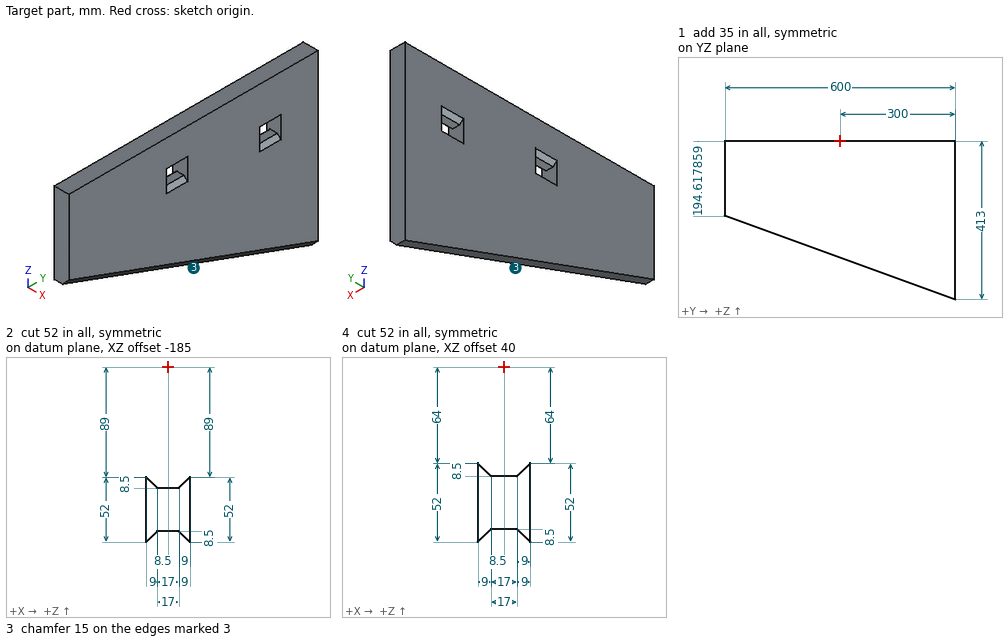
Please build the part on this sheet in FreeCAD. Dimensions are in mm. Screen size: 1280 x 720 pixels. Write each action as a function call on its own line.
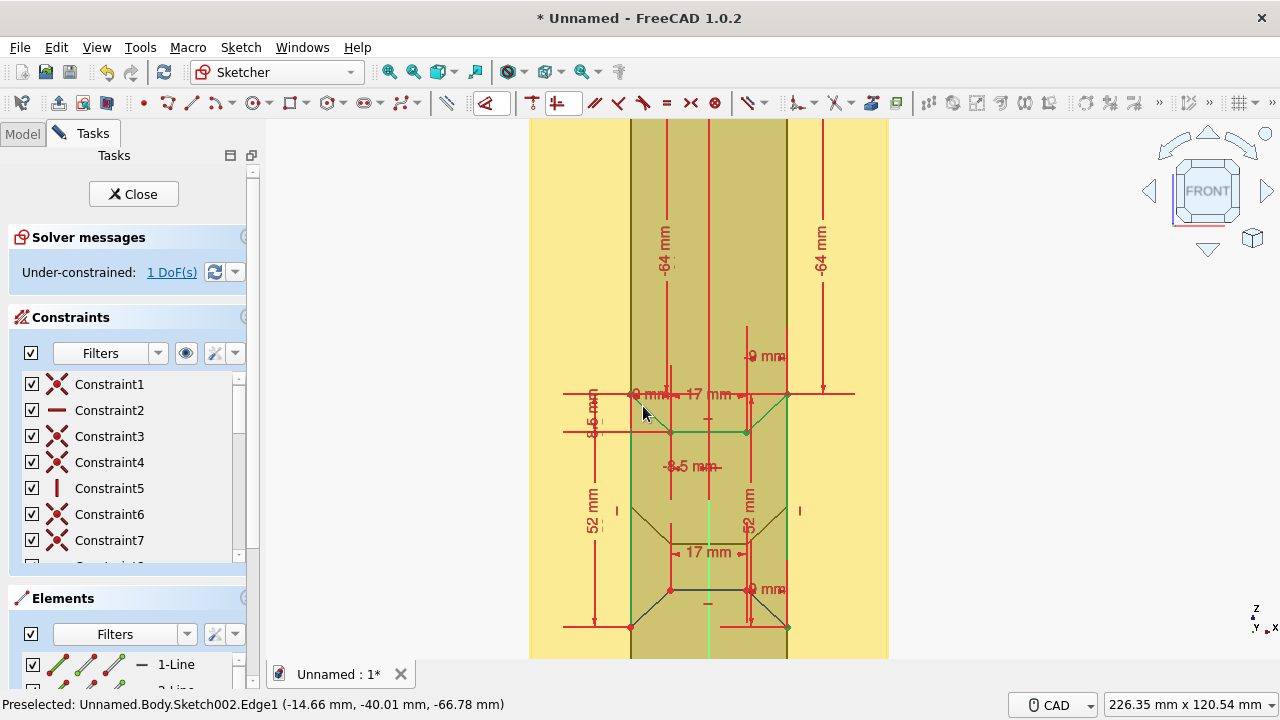
click(775, 616)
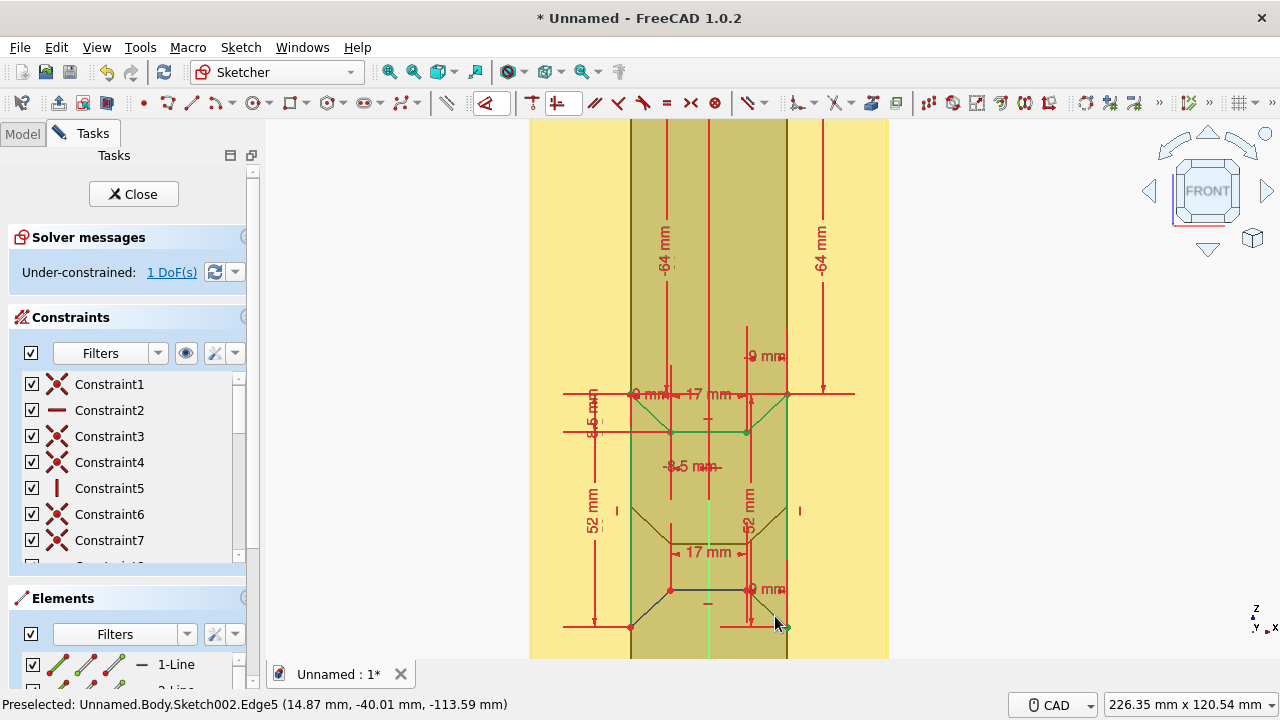
key(i)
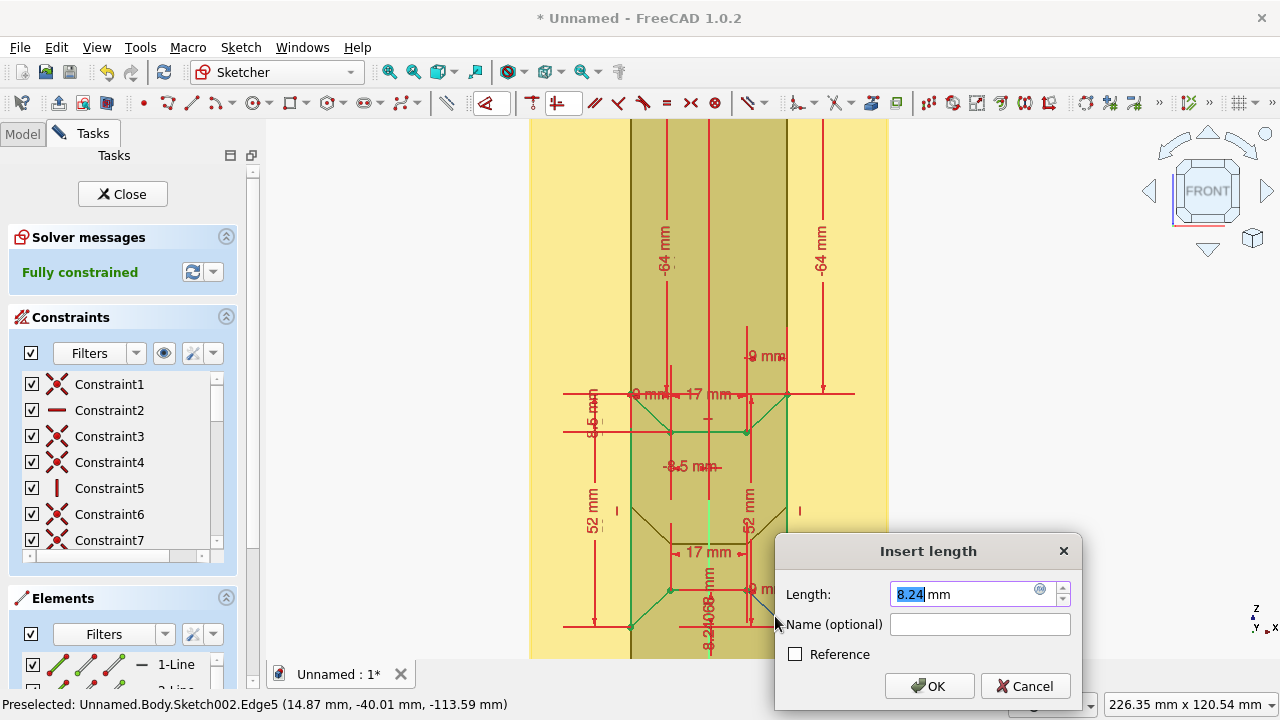
text(8.5)
key(Return)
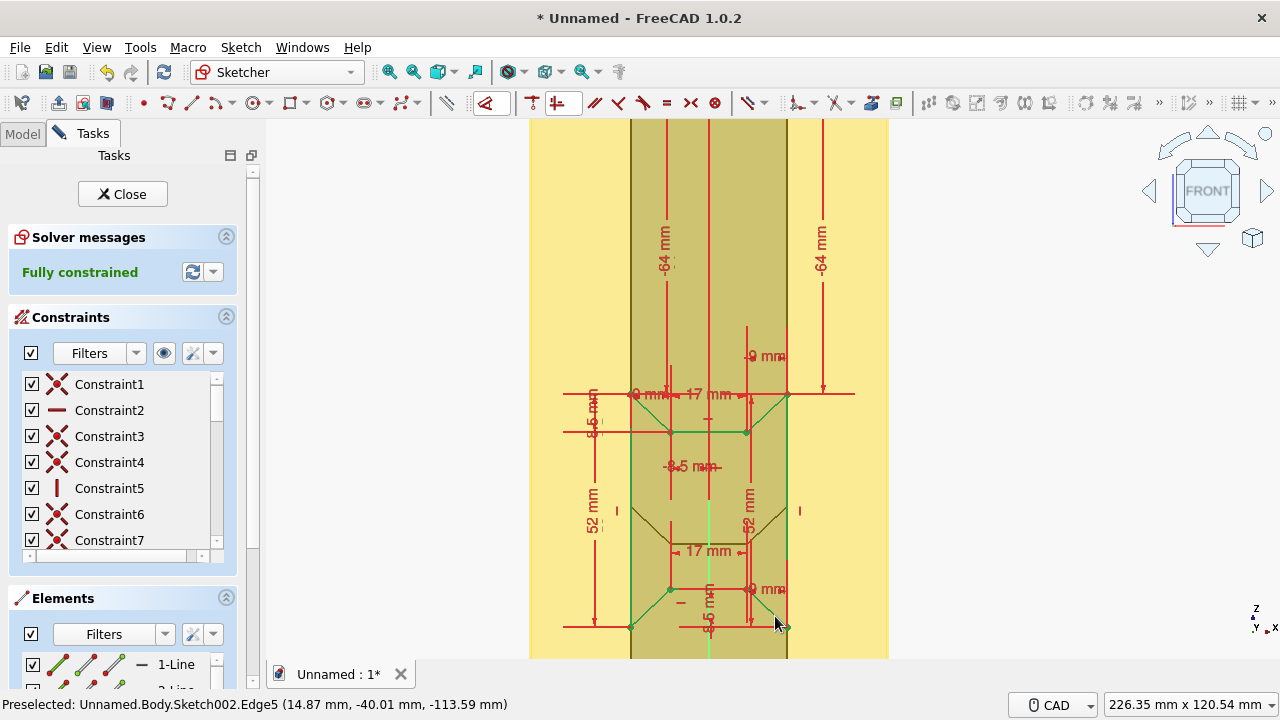
click(123, 194)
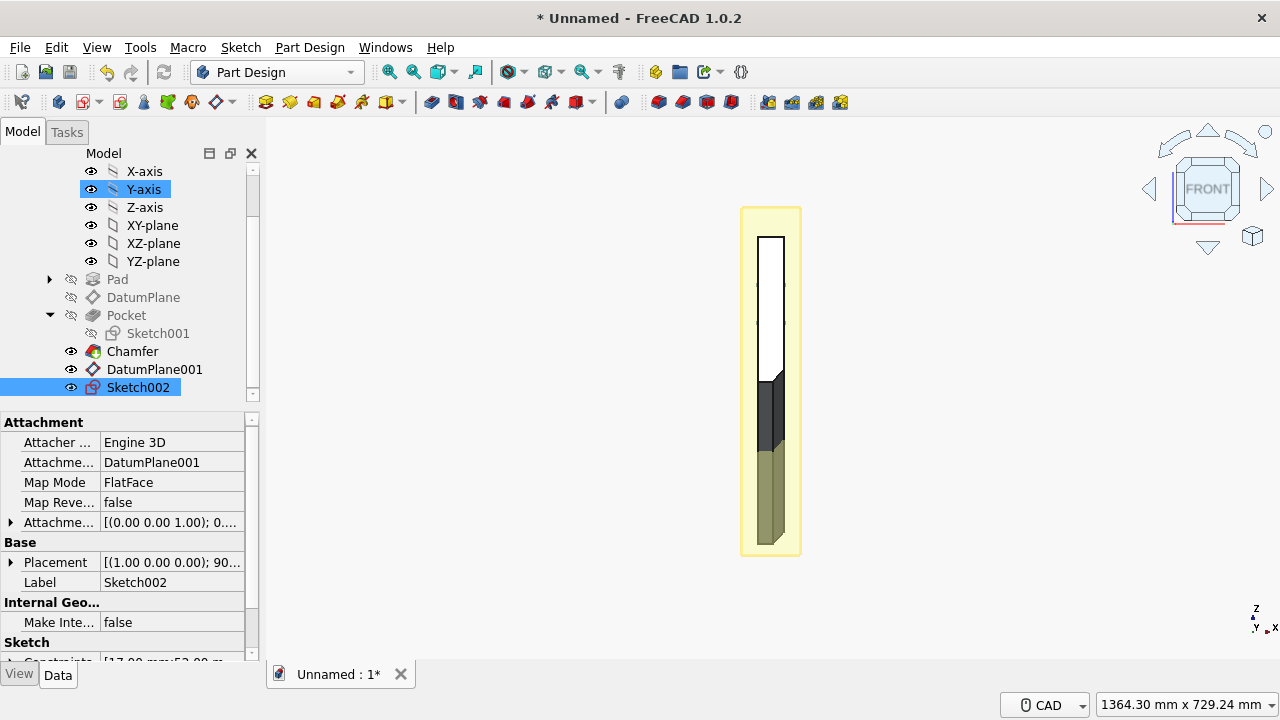
click(432, 102)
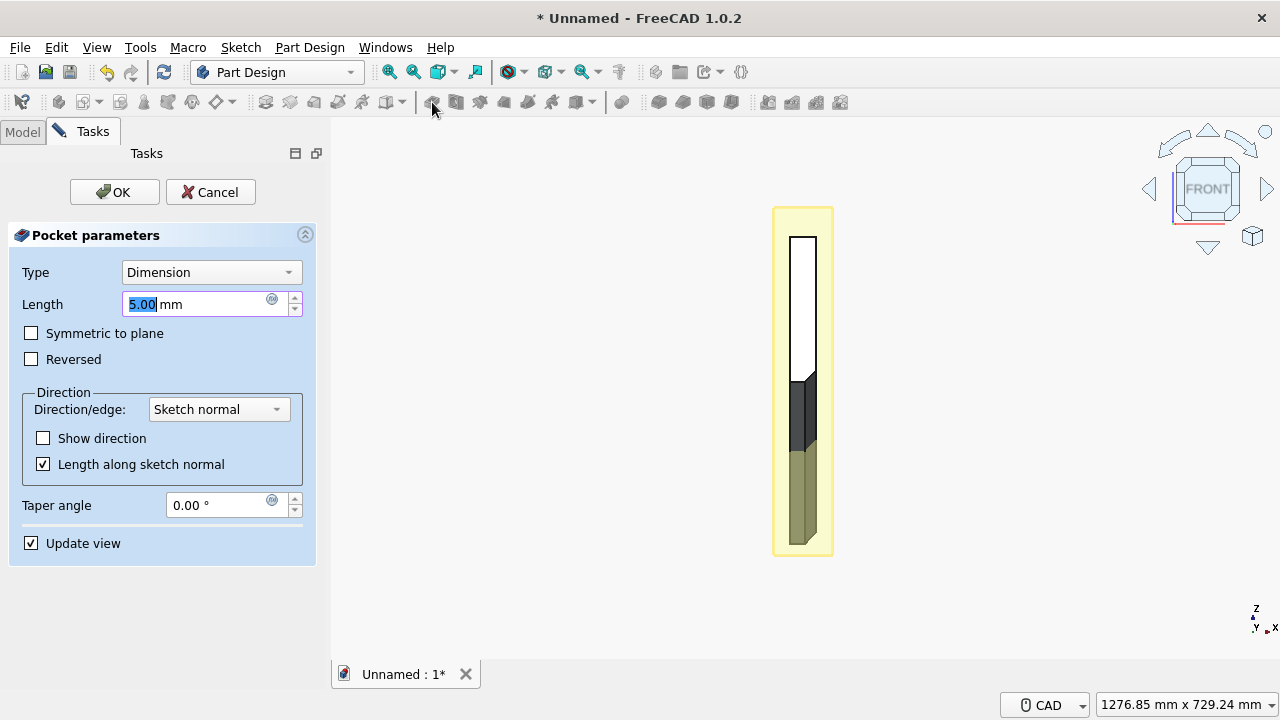
text(52)
key(Tab)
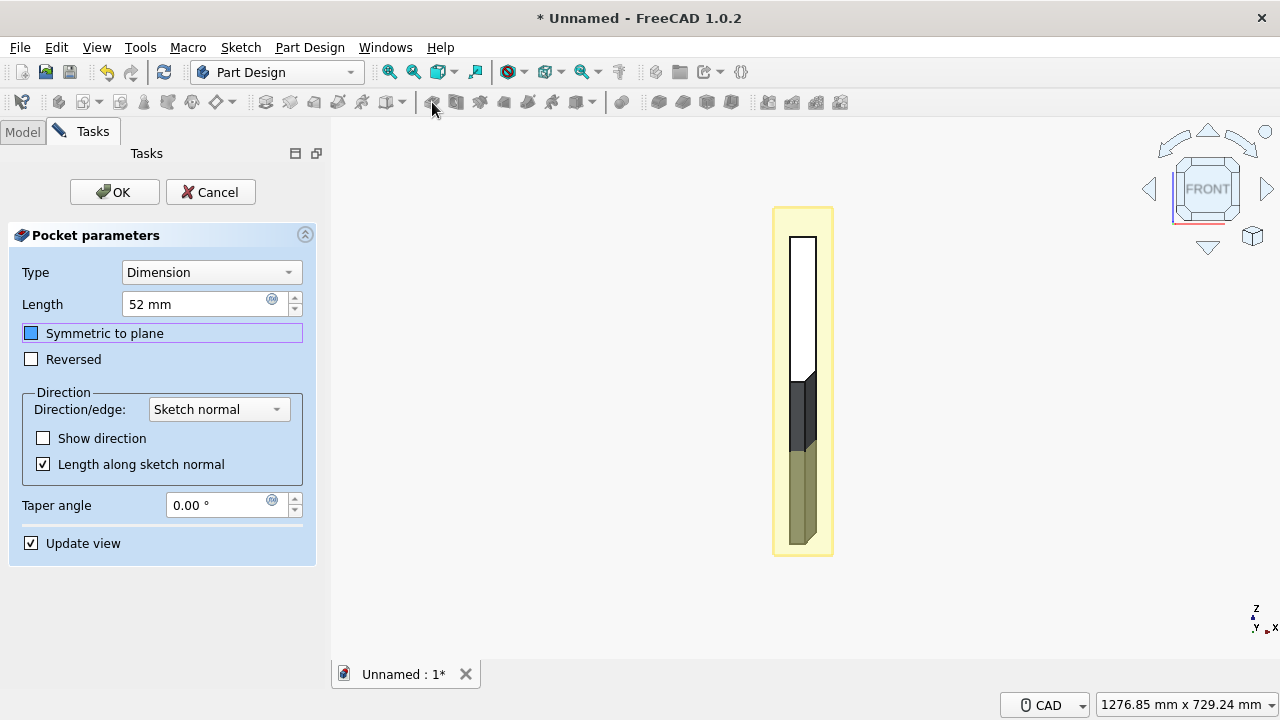
click(30, 333)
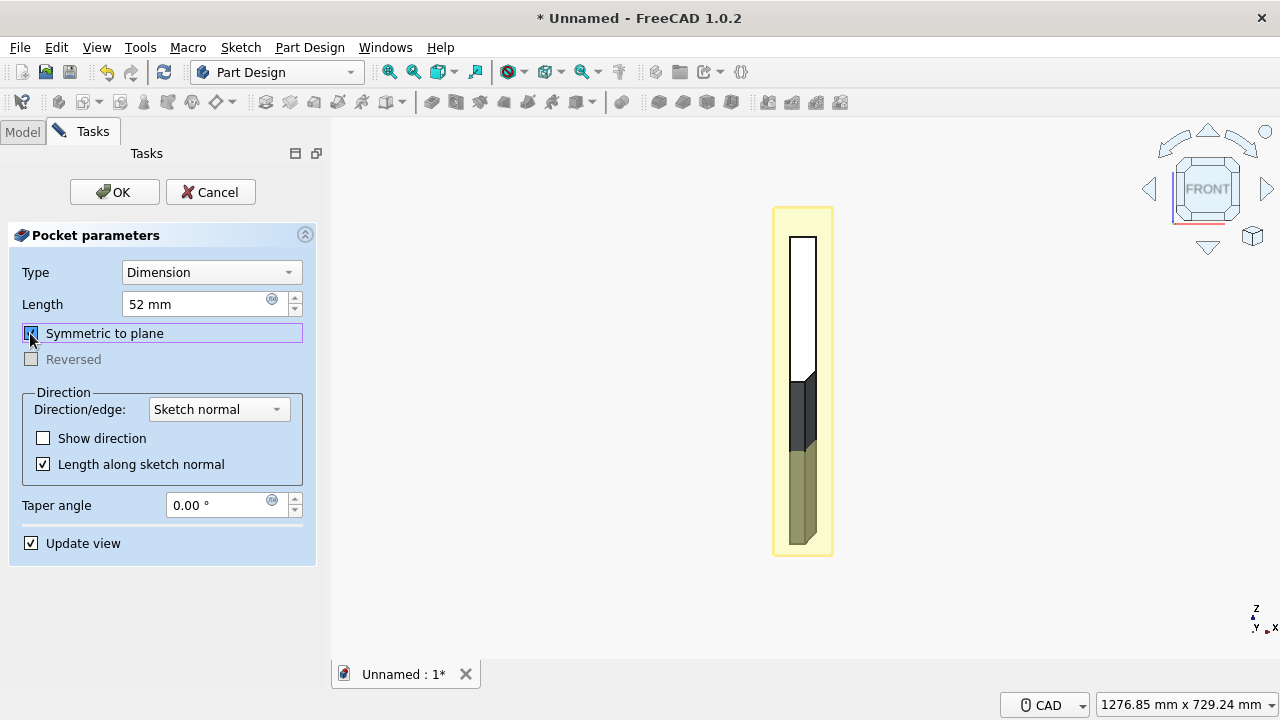
click(115, 192)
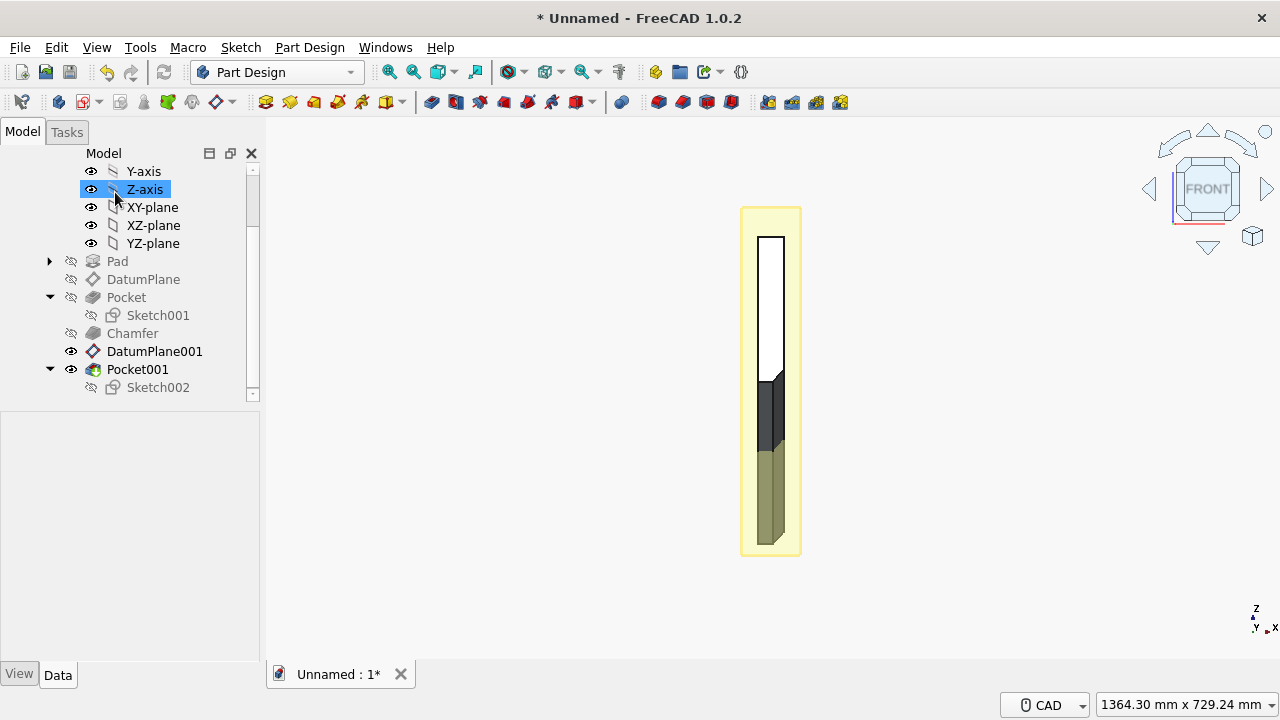
click(116, 351)
key(space)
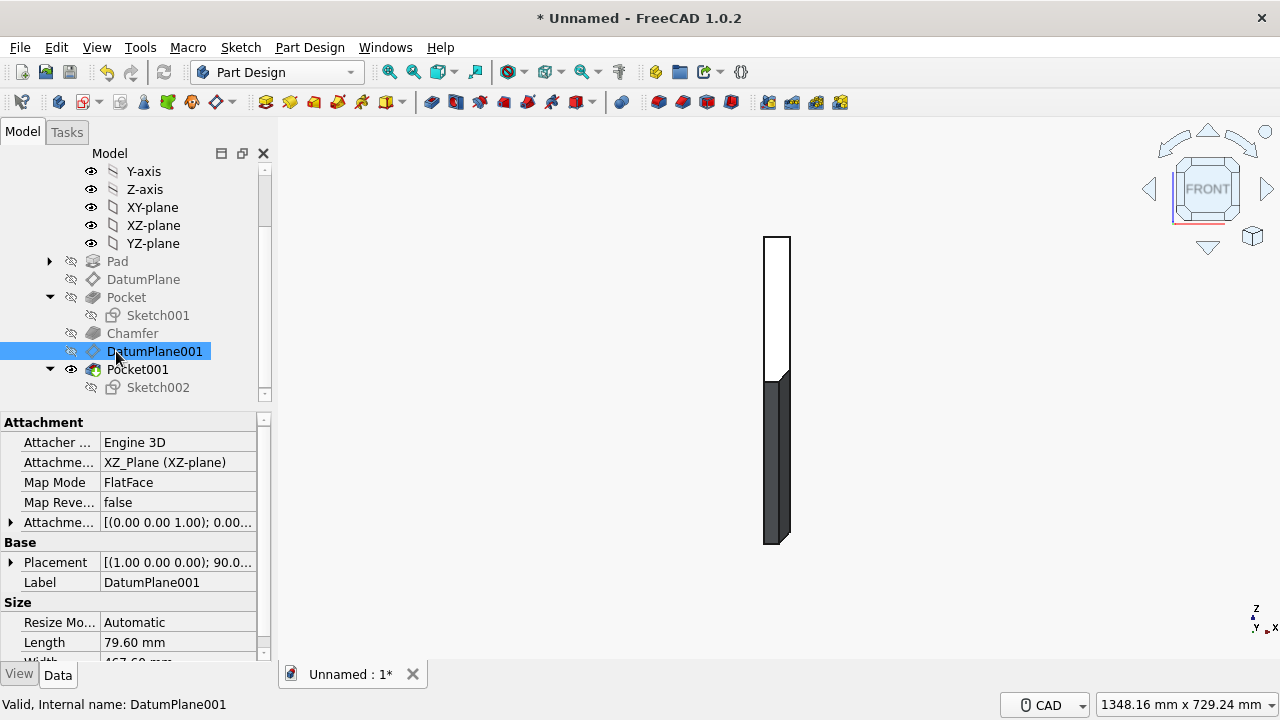
key(0)